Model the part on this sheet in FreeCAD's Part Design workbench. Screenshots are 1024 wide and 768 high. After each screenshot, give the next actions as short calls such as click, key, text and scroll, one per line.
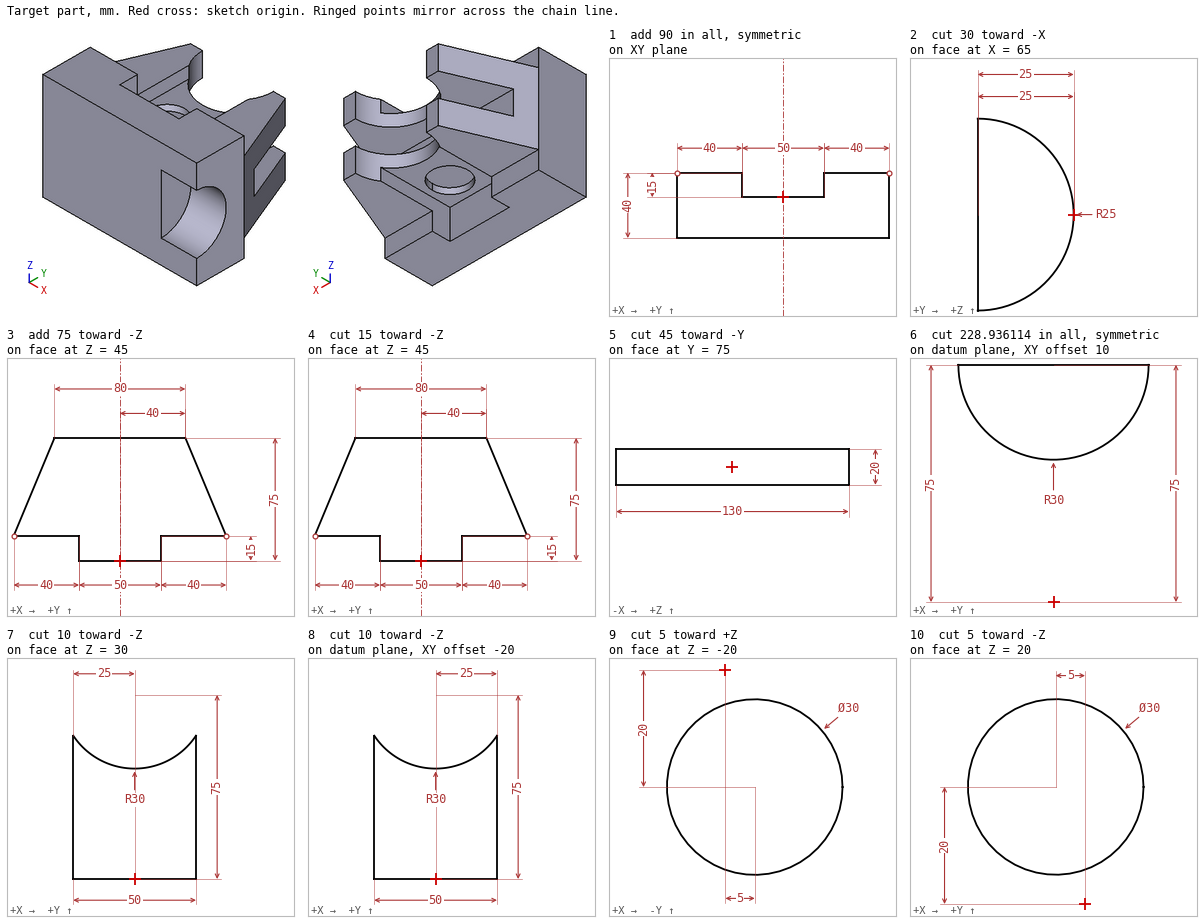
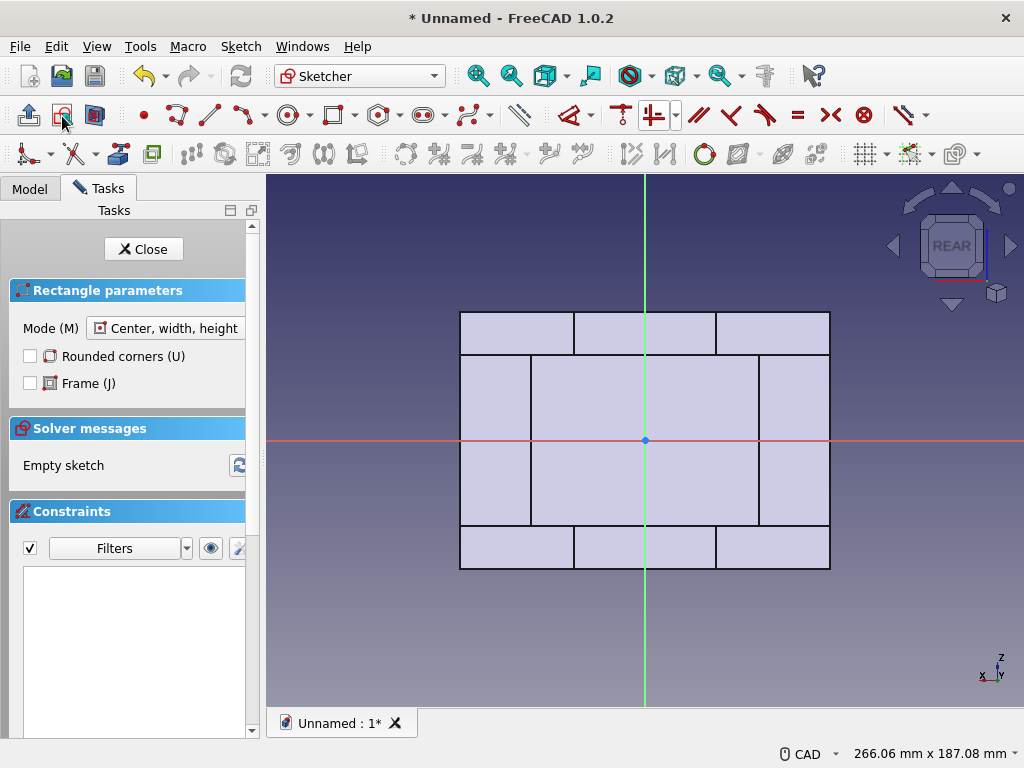
click(645, 440)
click(830, 412)
key(Escape)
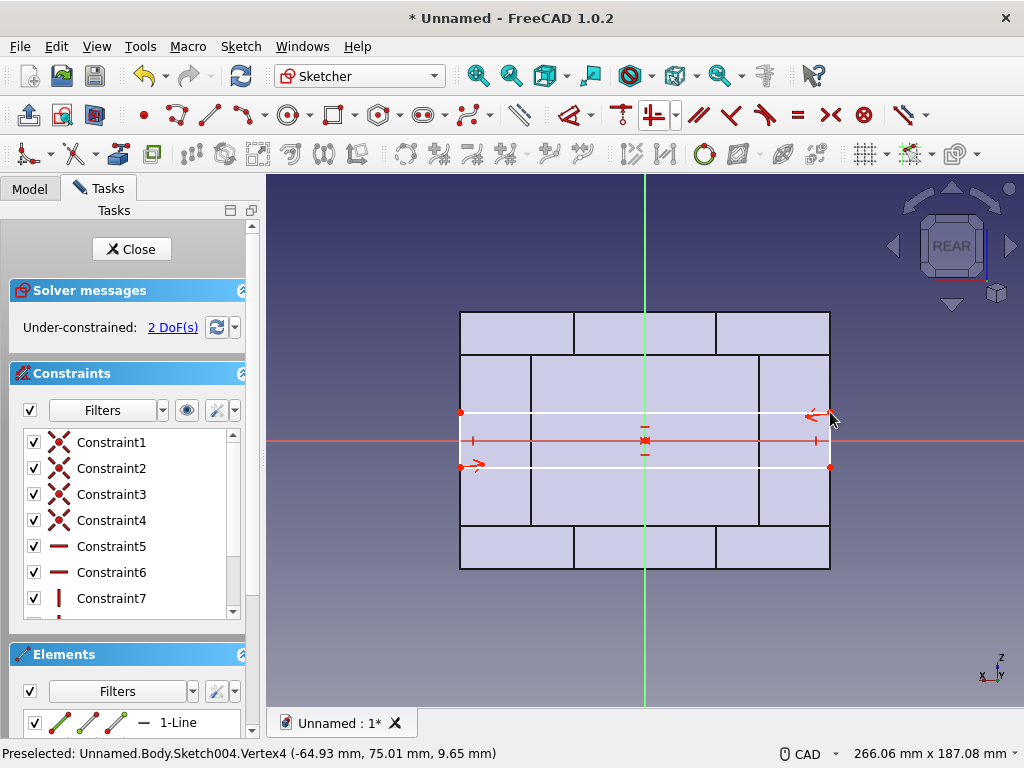
key(d)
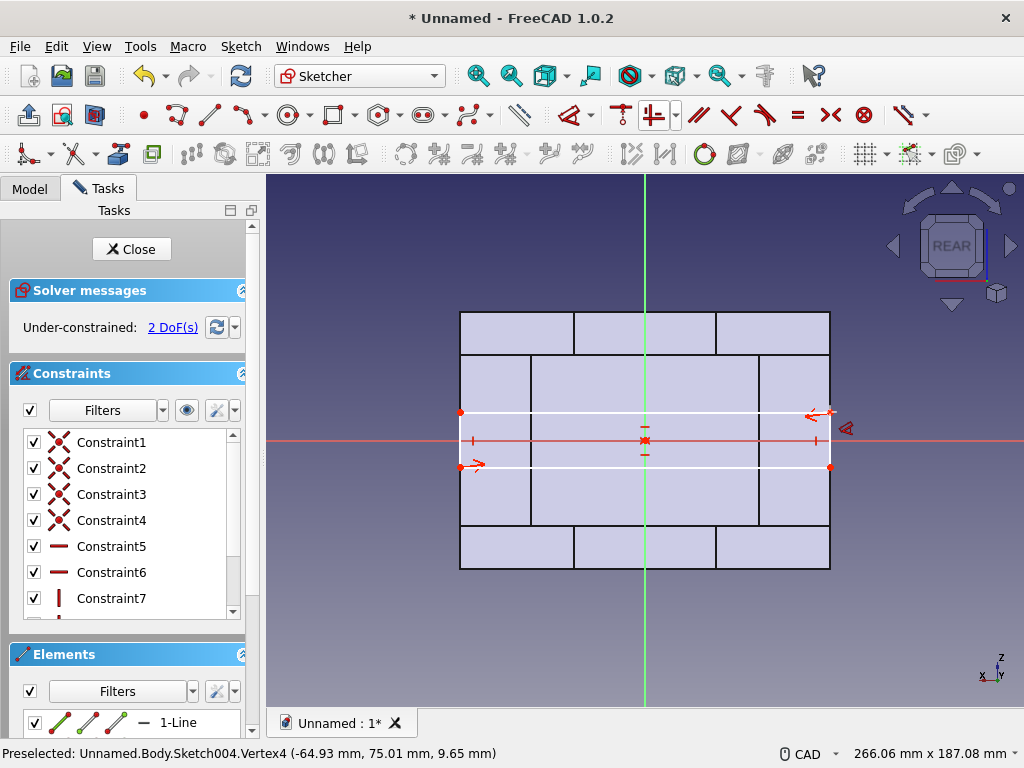
scroll(830, 451, up, 2)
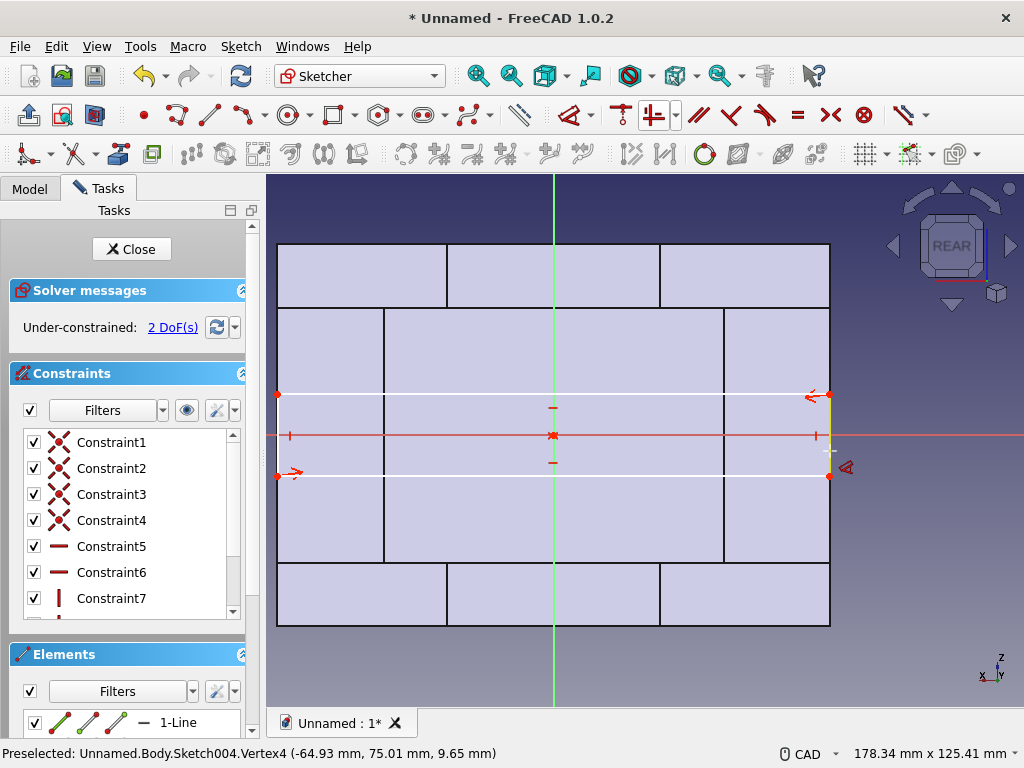
click(830, 451)
click(796, 416)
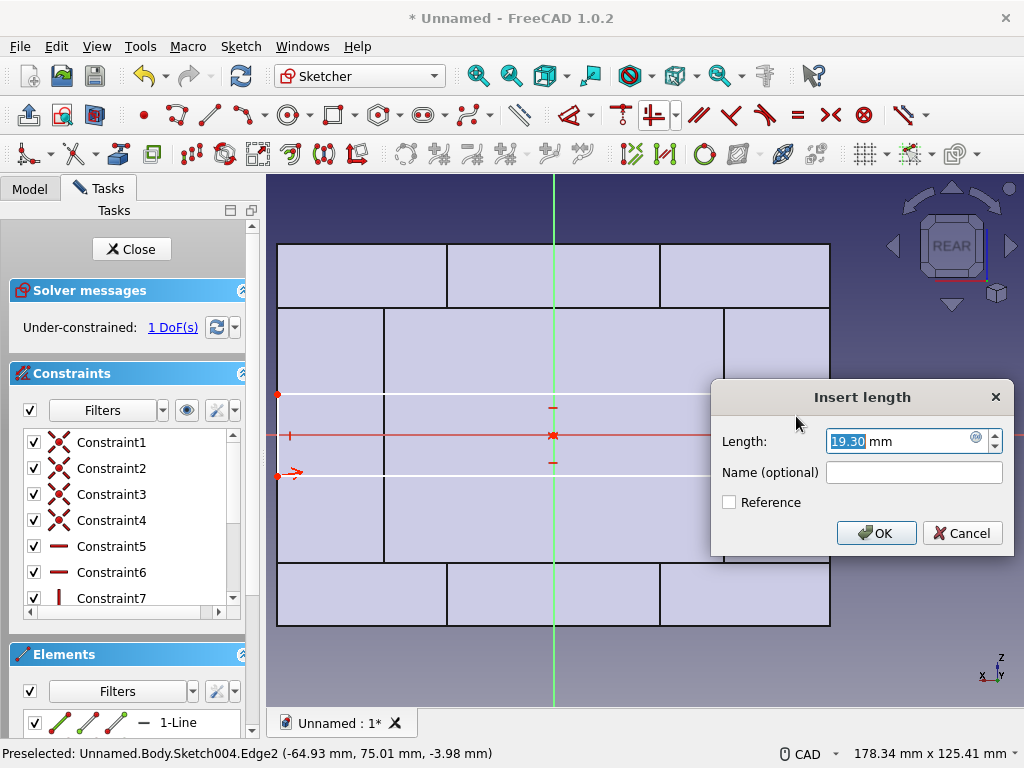
text(20)
key(Return)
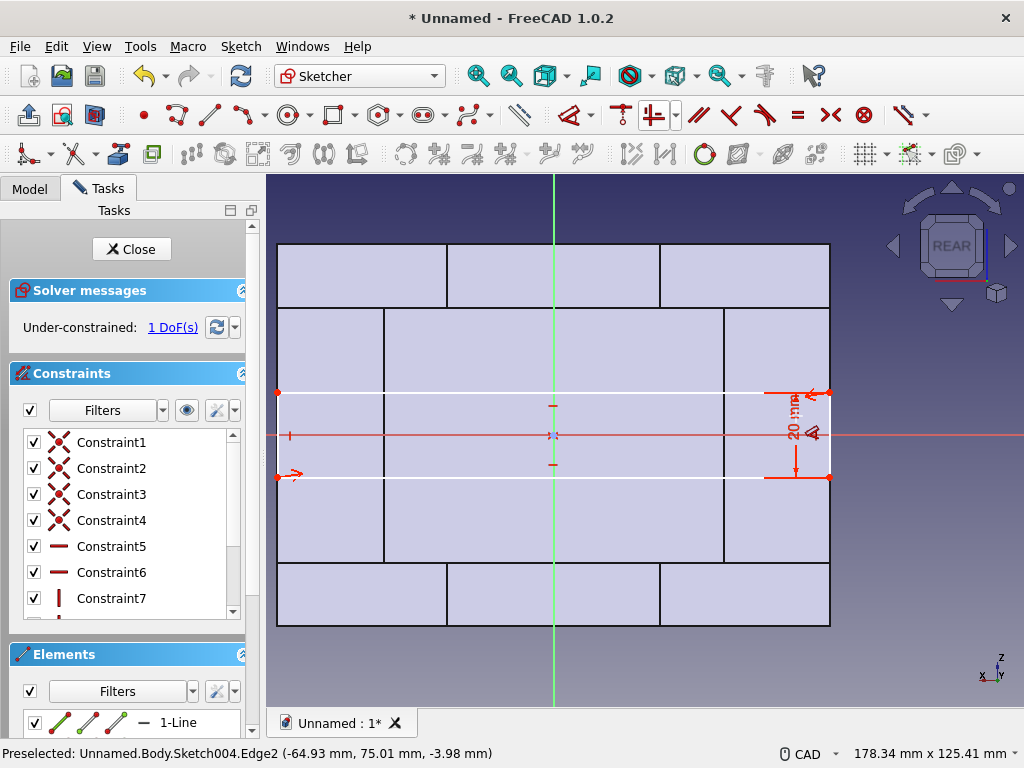
click(443, 478)
click(439, 512)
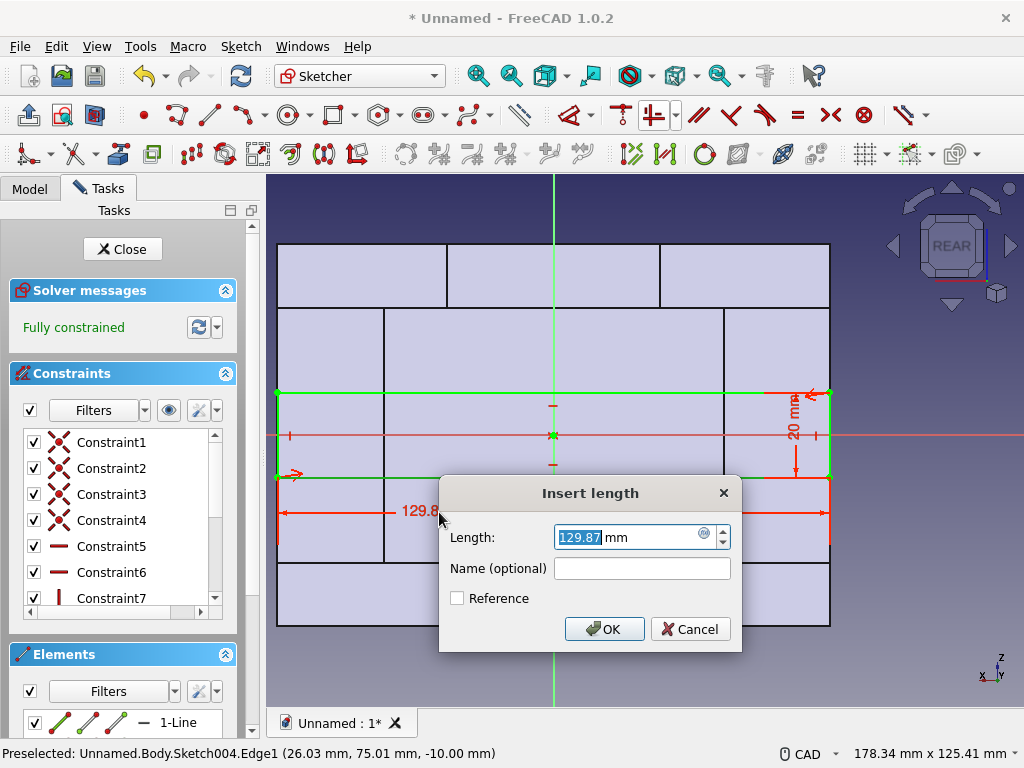
text(130)
key(Return)
key(Escape)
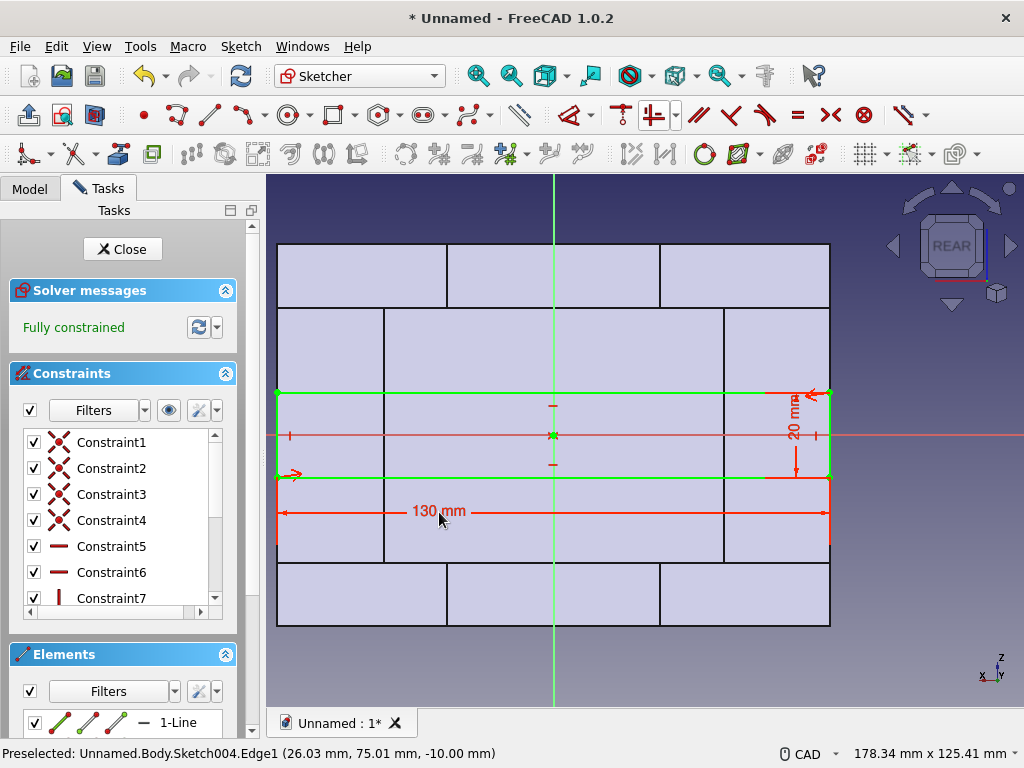
click(123, 249)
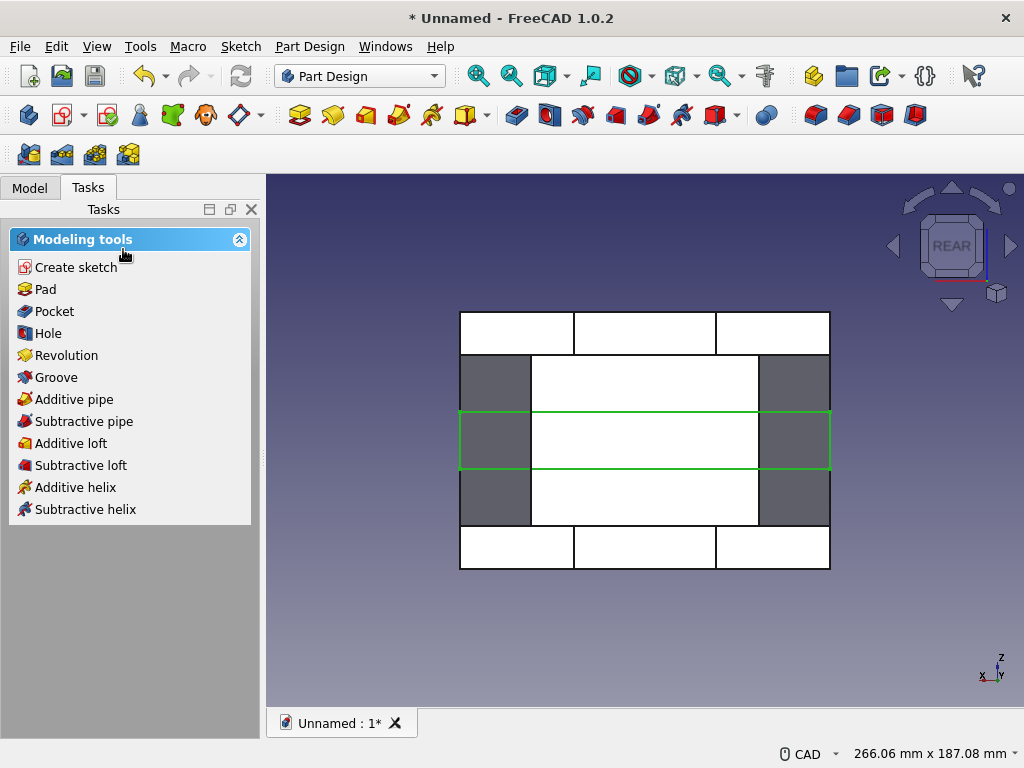
click(517, 116)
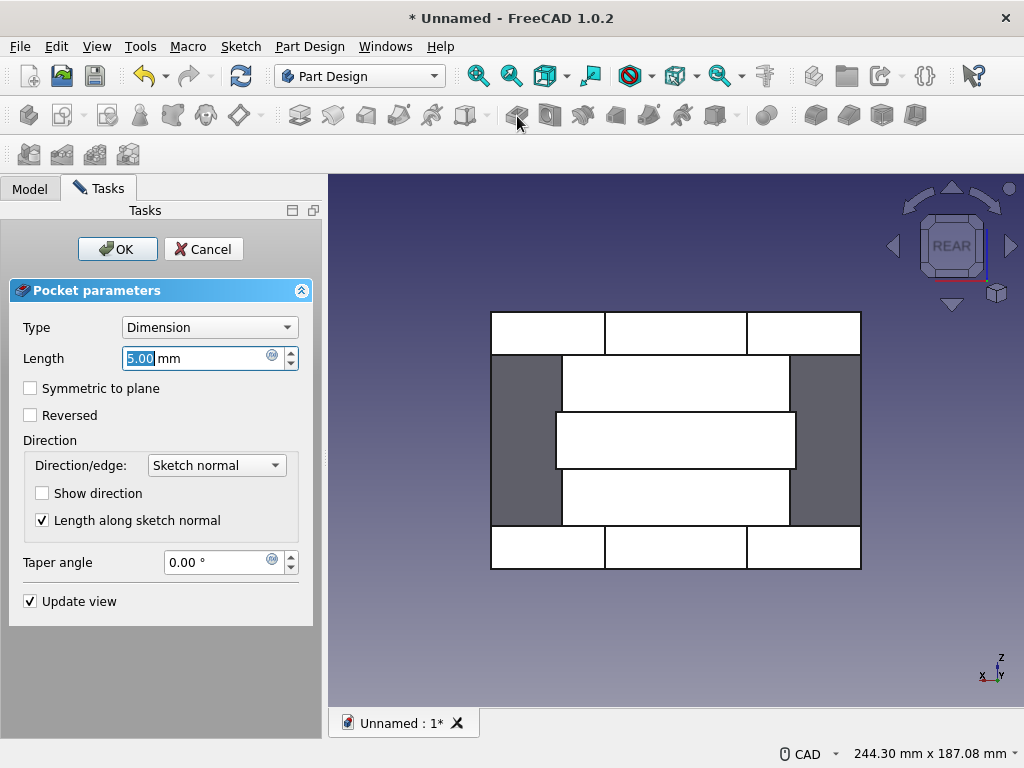
text(45)
key(Tab)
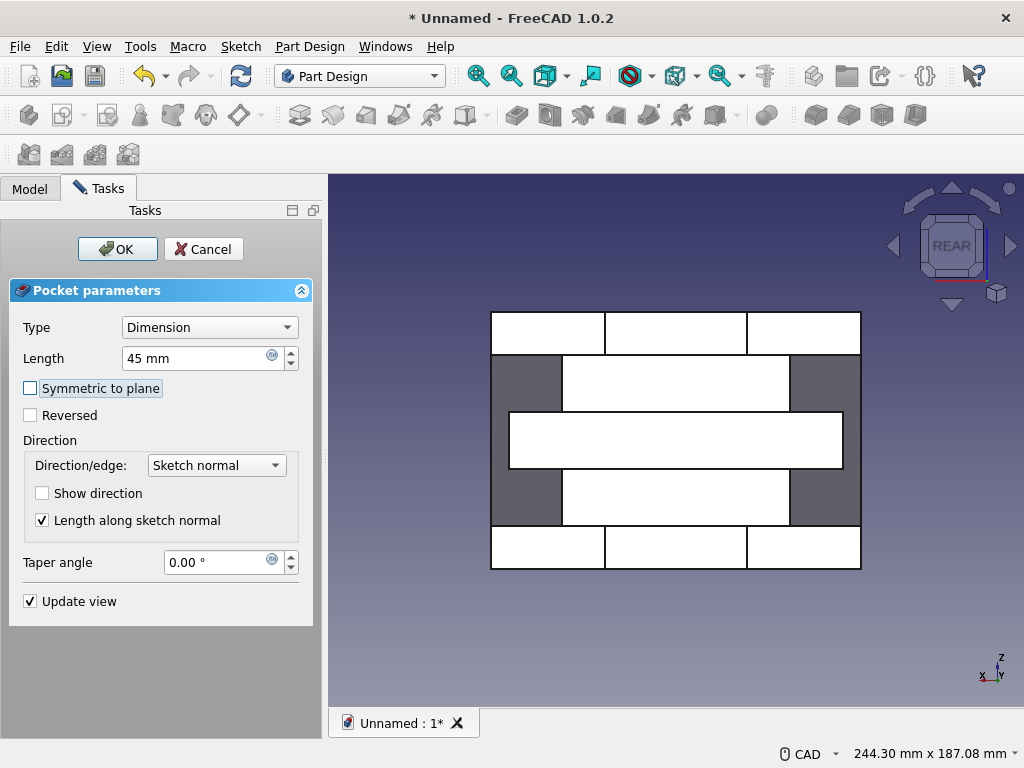
click(118, 249)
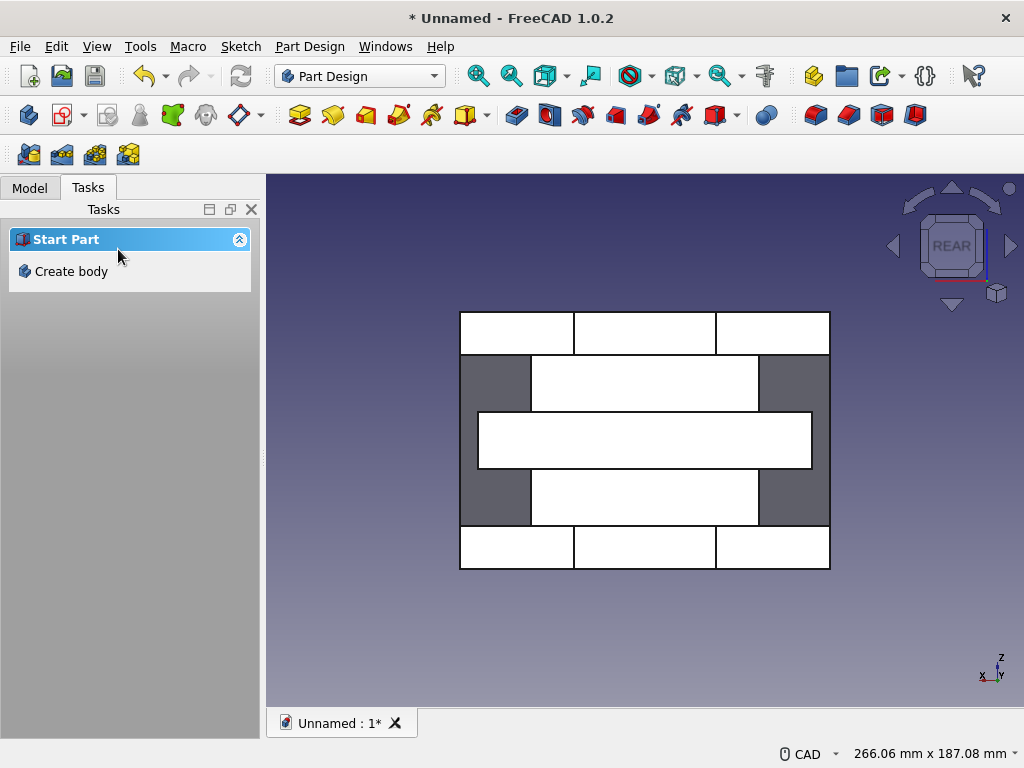
click(30, 188)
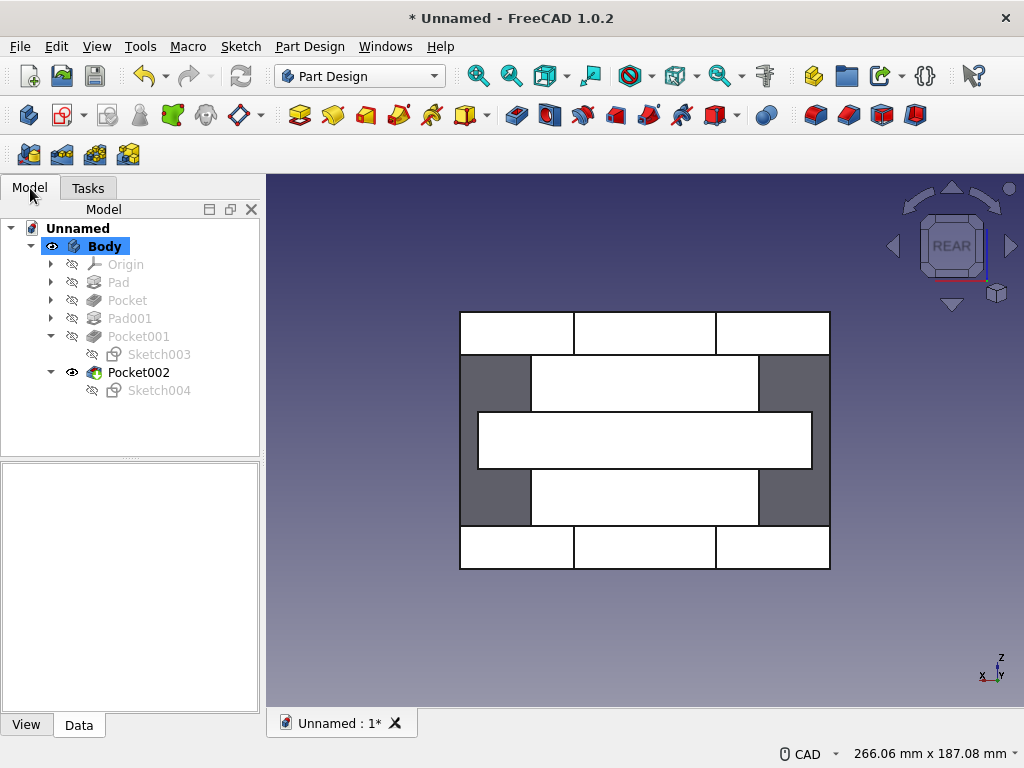
click(51, 264)